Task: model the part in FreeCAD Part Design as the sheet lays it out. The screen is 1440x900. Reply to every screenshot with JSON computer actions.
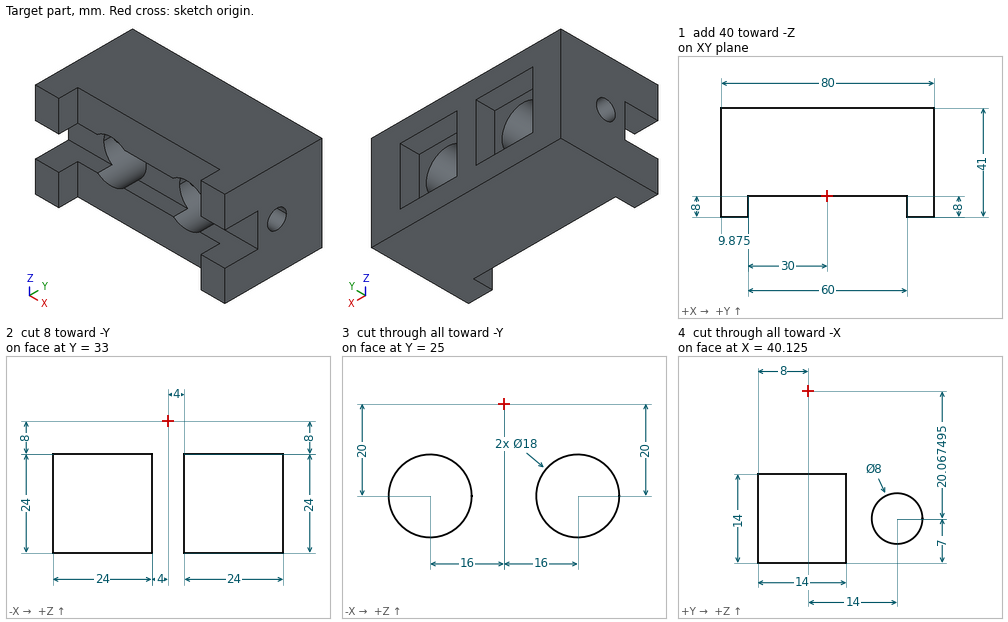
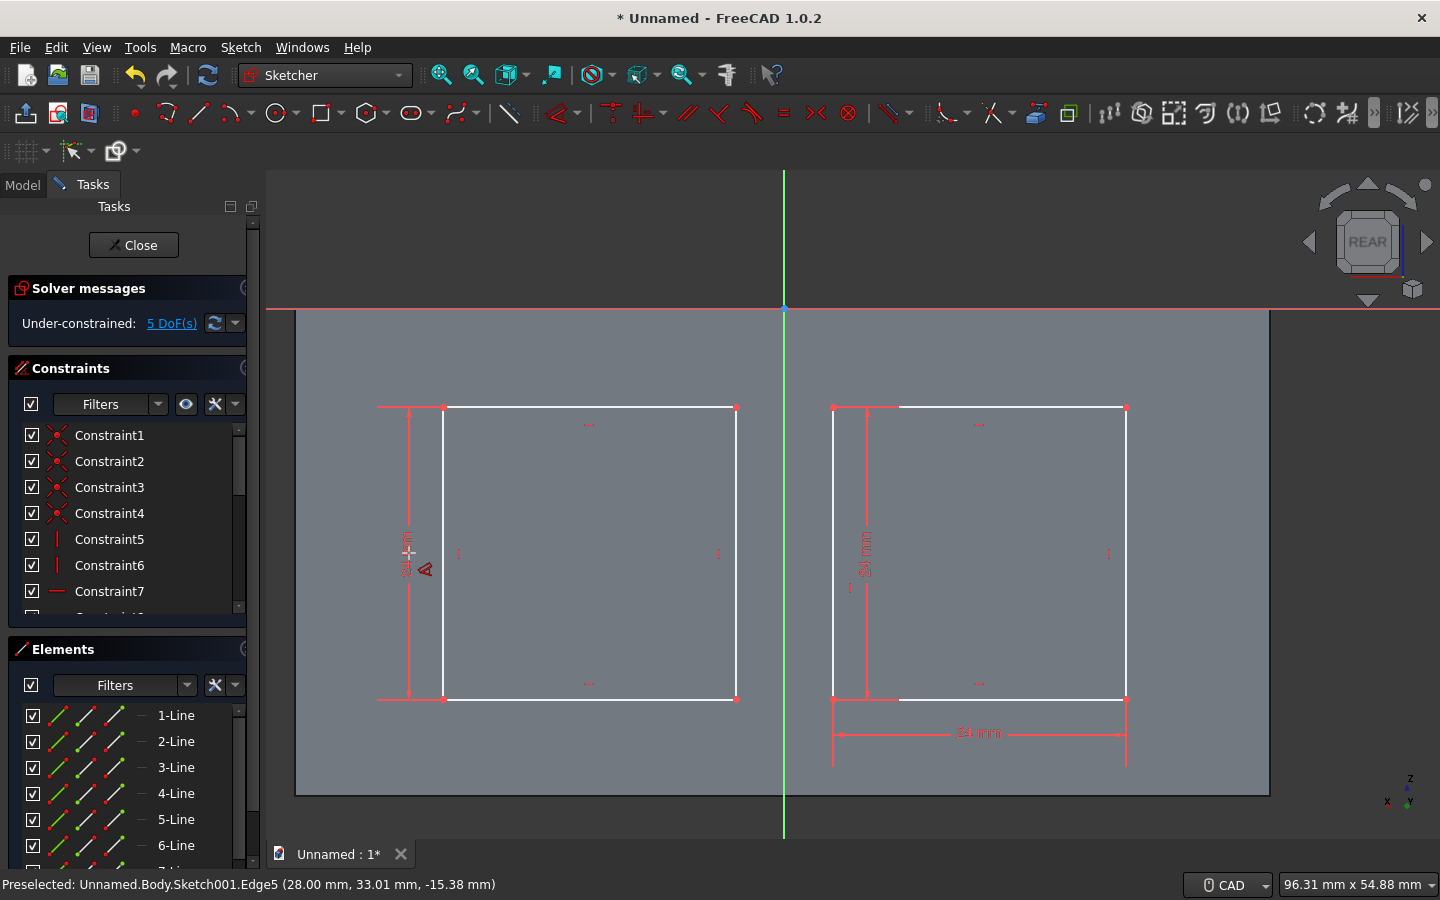
{"action": "left_click", "coordinate": [531, 700]}
{"action": "left_click", "coordinate": [590, 734]}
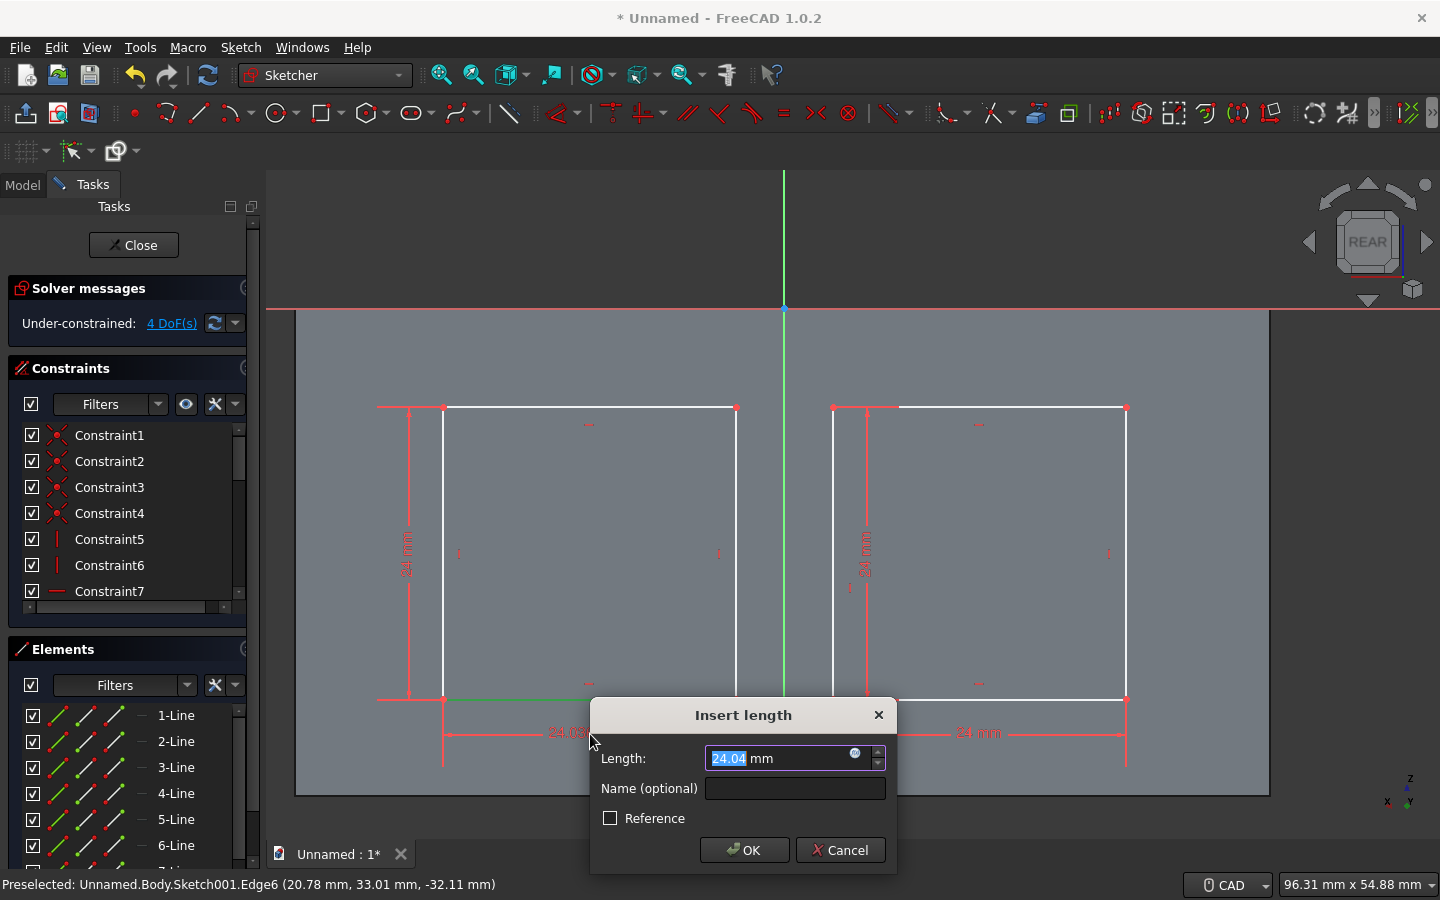
{"action": "type", "text": "24"}
{"action": "key", "text": "Return"}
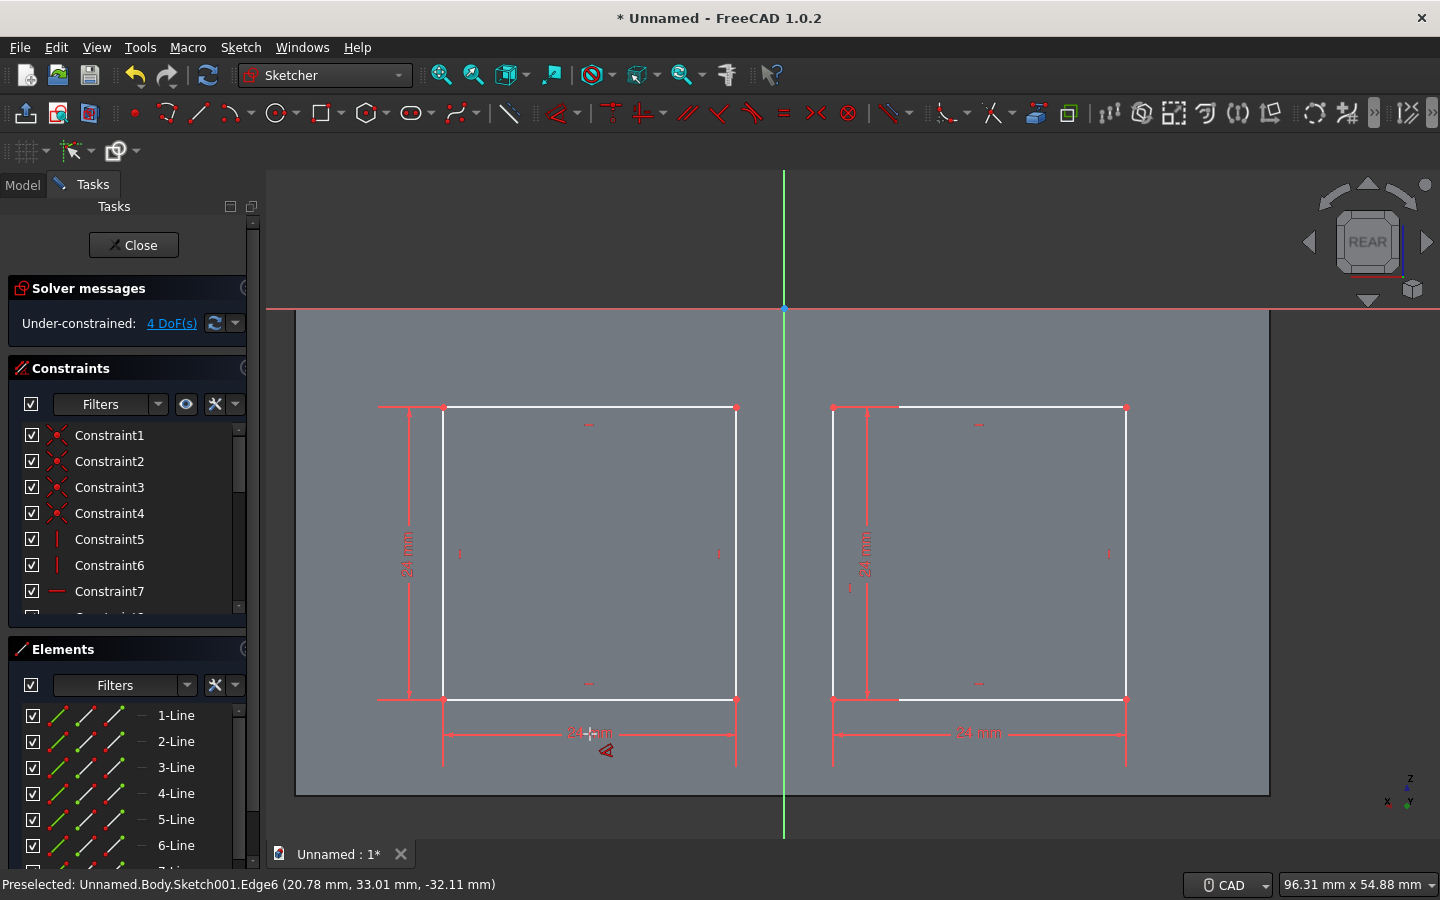
{"action": "left_click", "coordinate": [833, 407]}
{"action": "left_click", "coordinate": [809, 275]}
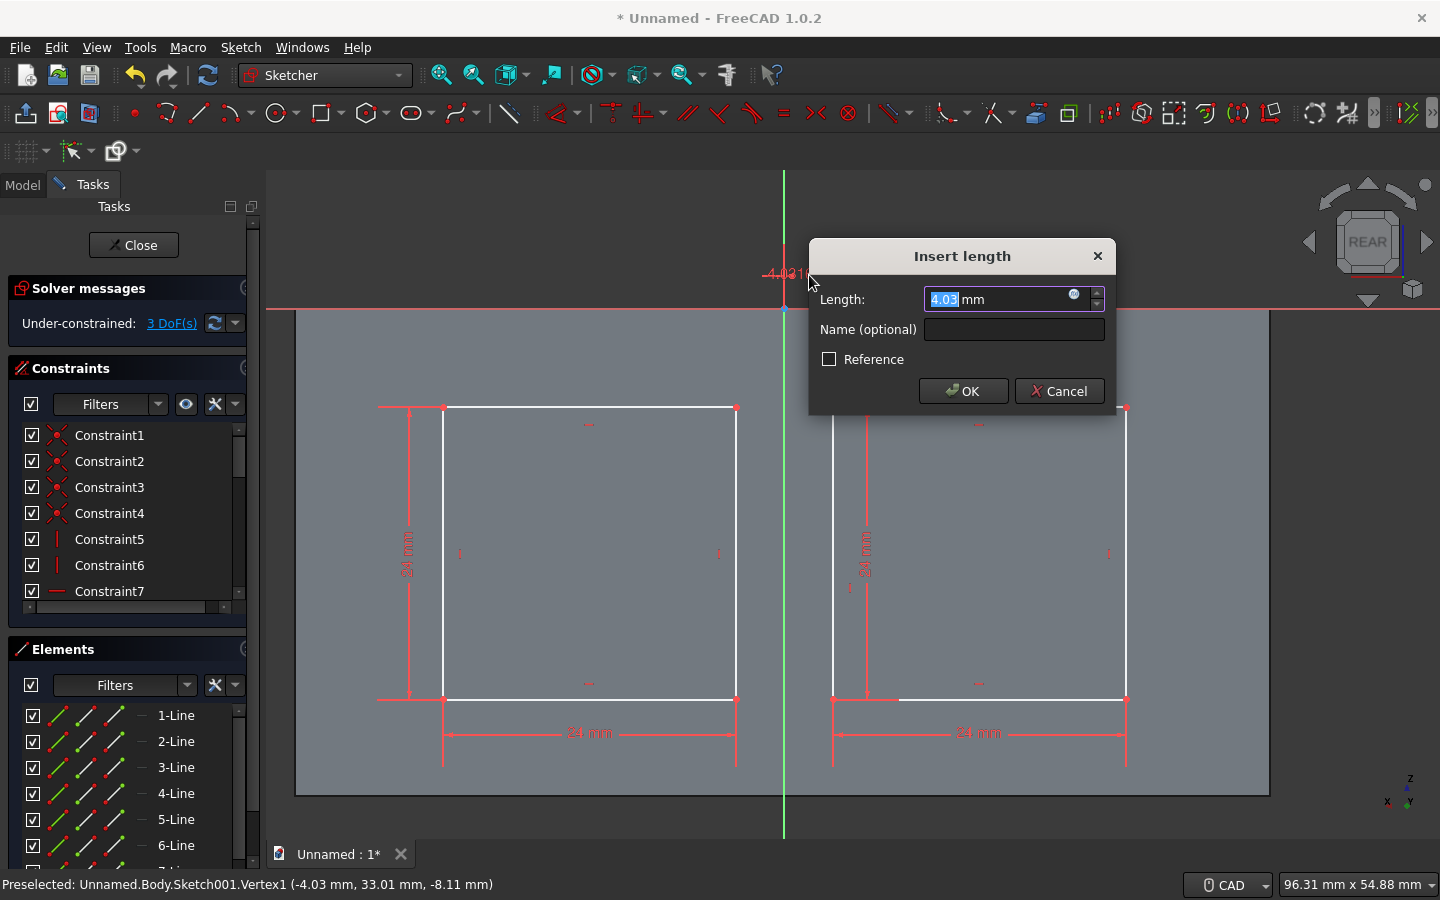
{"action": "type", "text": "4"}
{"action": "key", "text": "Return"}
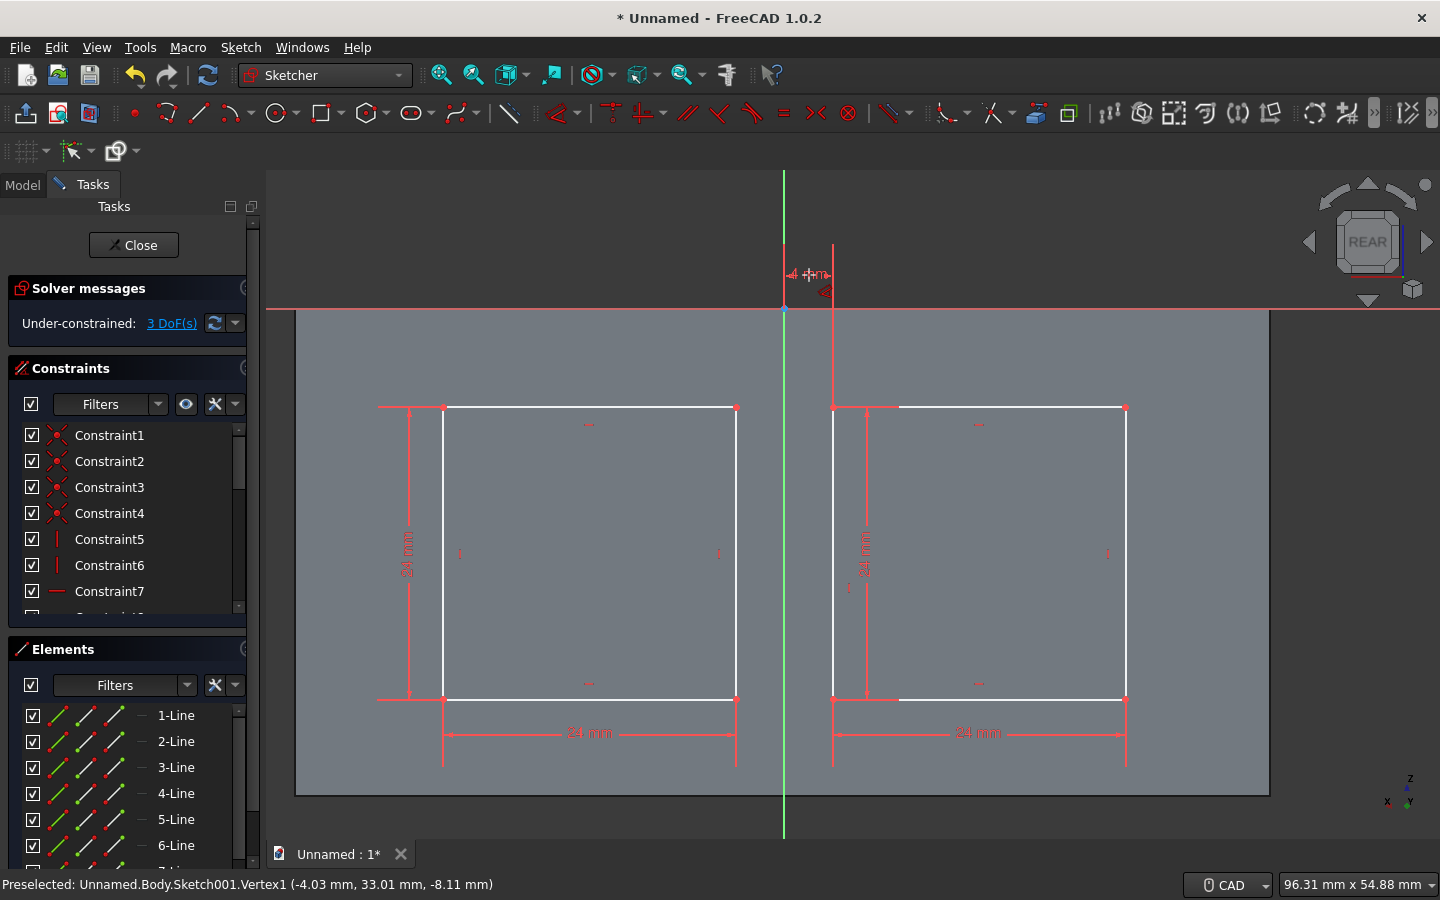
{"action": "left_click", "coordinate": [833, 407]}
{"action": "left_click", "coordinate": [867, 358]}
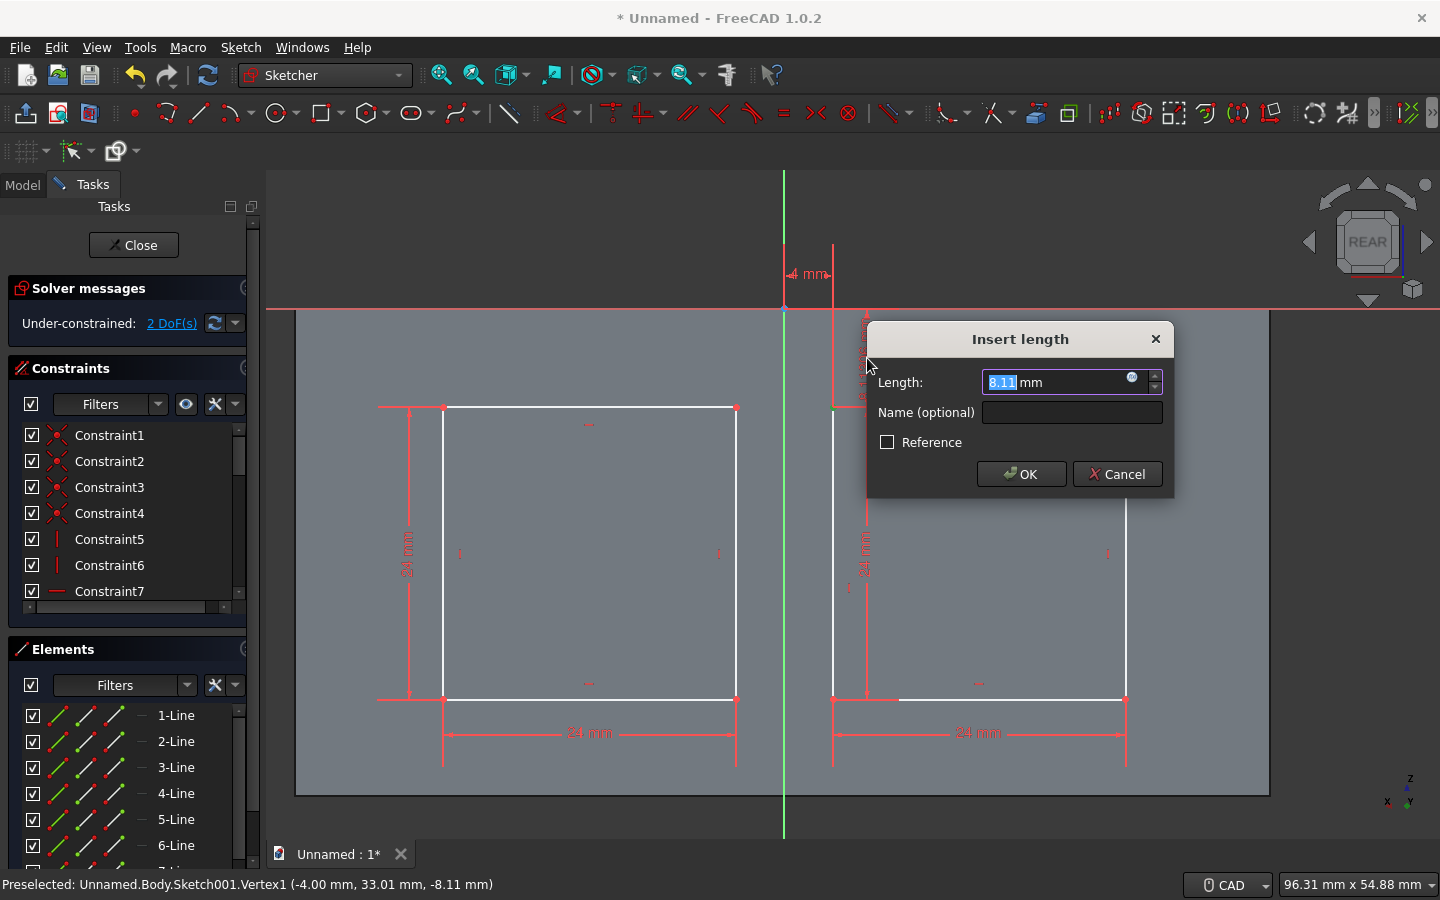
{"action": "type", "text": "8"}
{"action": "key", "text": "Return"}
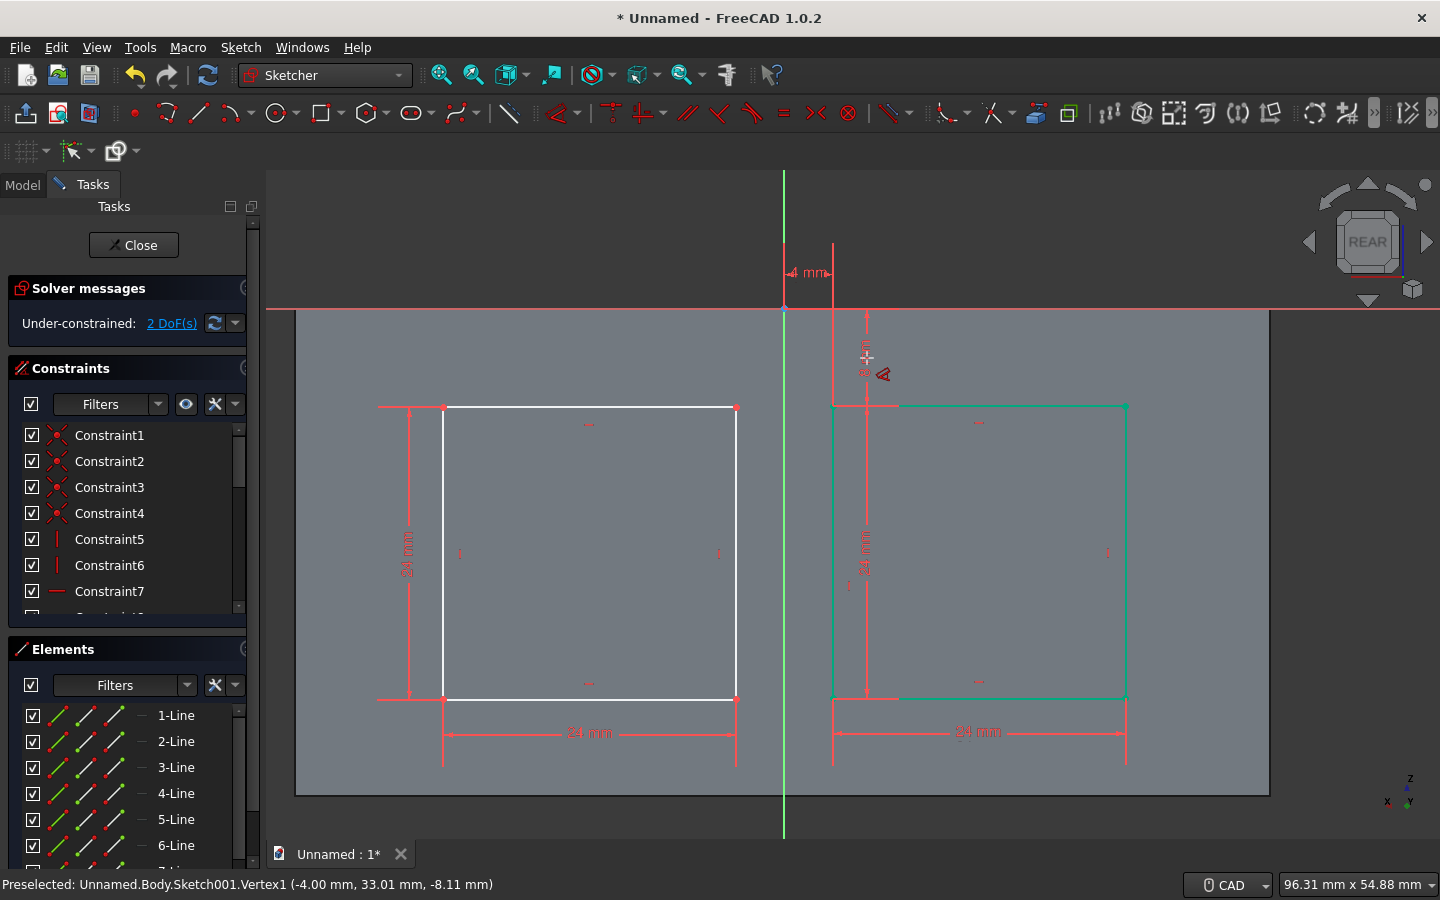
{"action": "left_click", "coordinate": [443, 407]}
{"action": "left_click", "coordinate": [409, 358]}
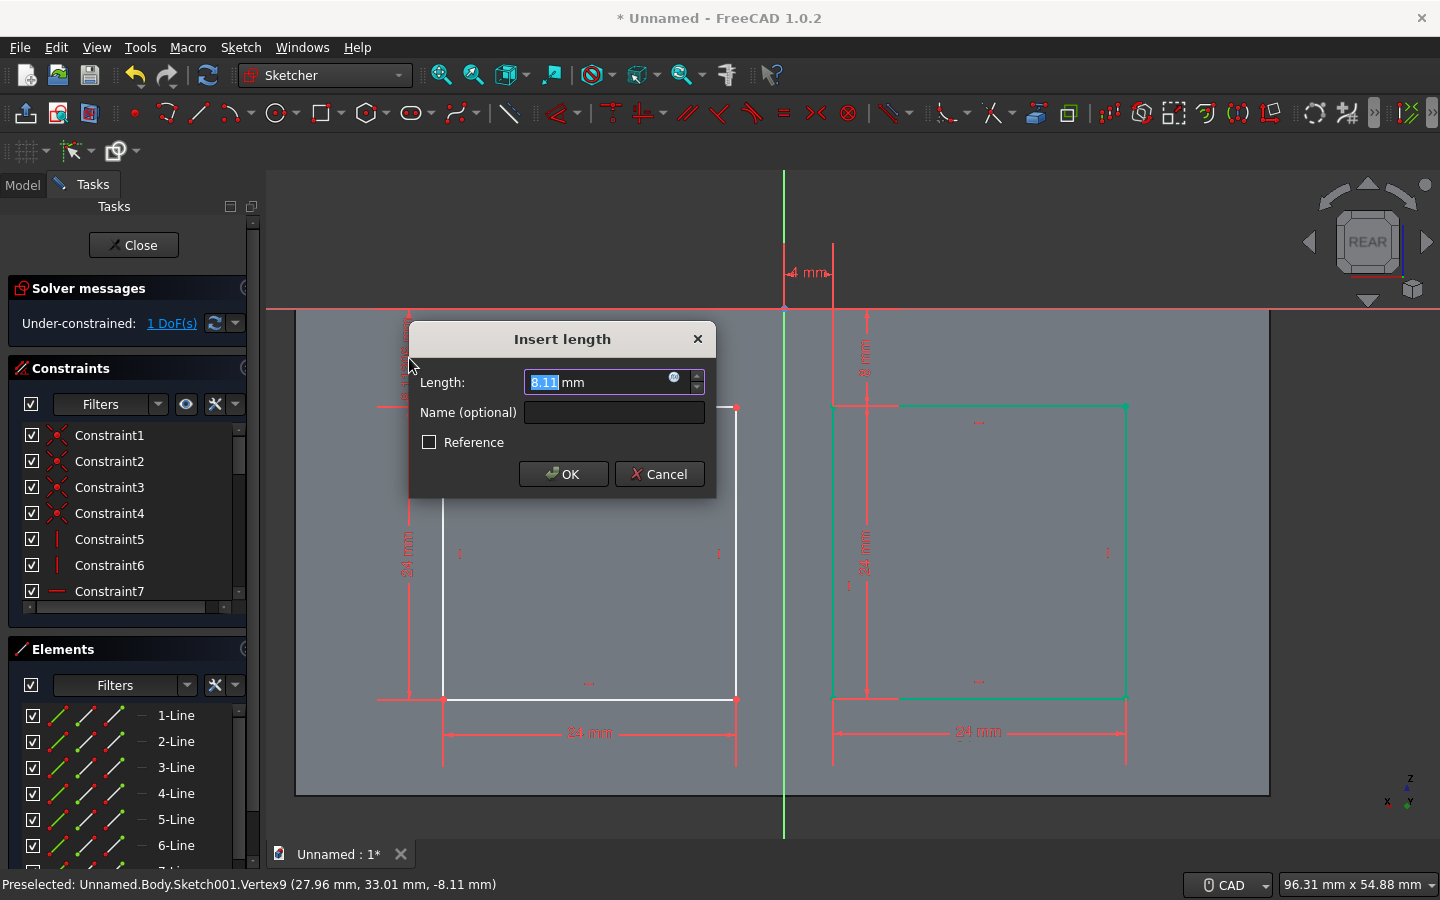
{"action": "type", "text": "8"}
{"action": "key", "text": "Return"}